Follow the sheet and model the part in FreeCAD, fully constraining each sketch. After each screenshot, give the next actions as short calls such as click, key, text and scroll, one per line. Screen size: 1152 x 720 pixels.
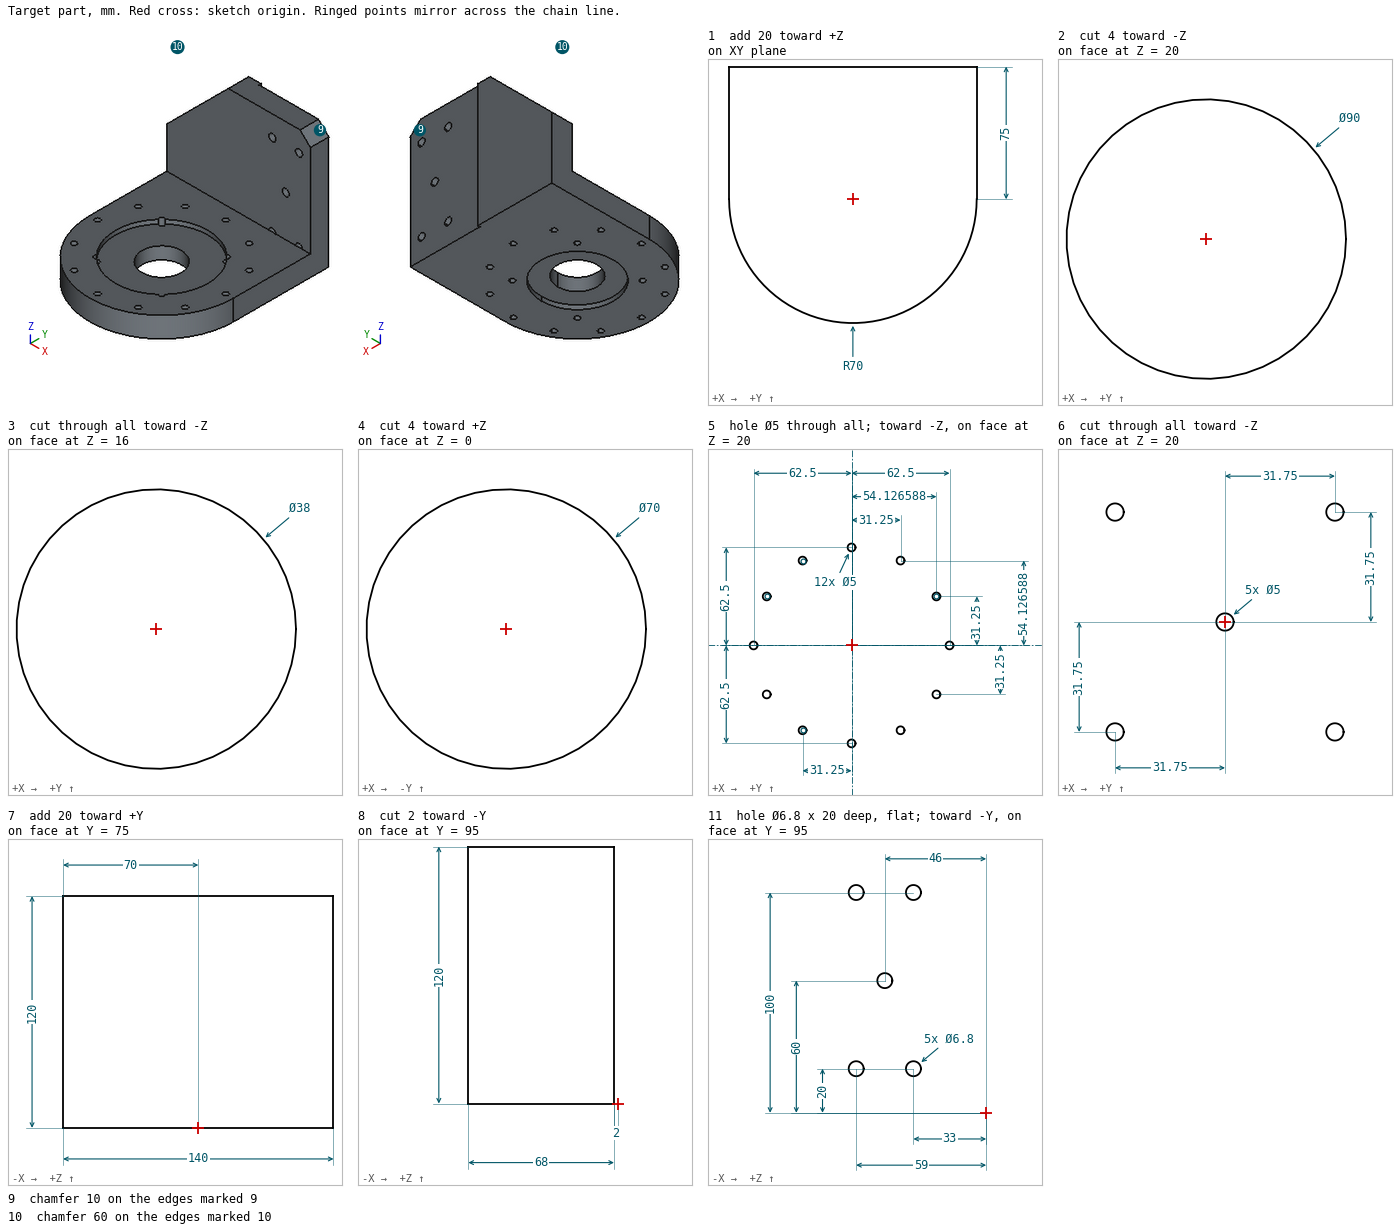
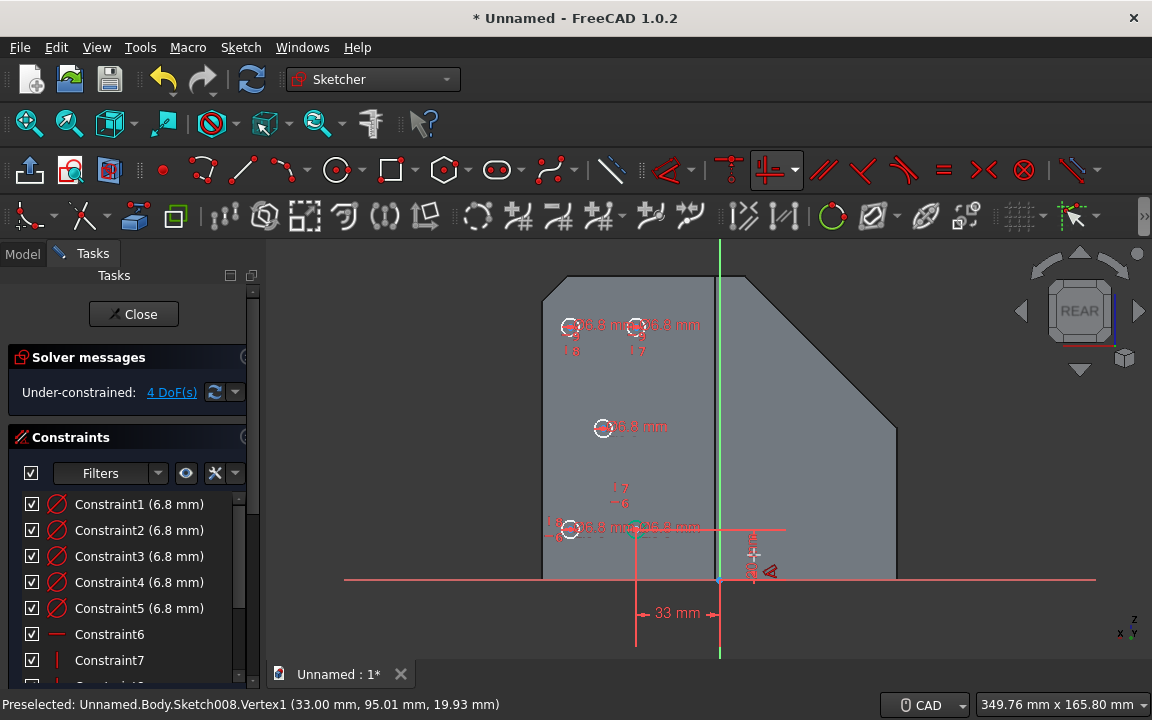
click(570, 530)
click(593, 614)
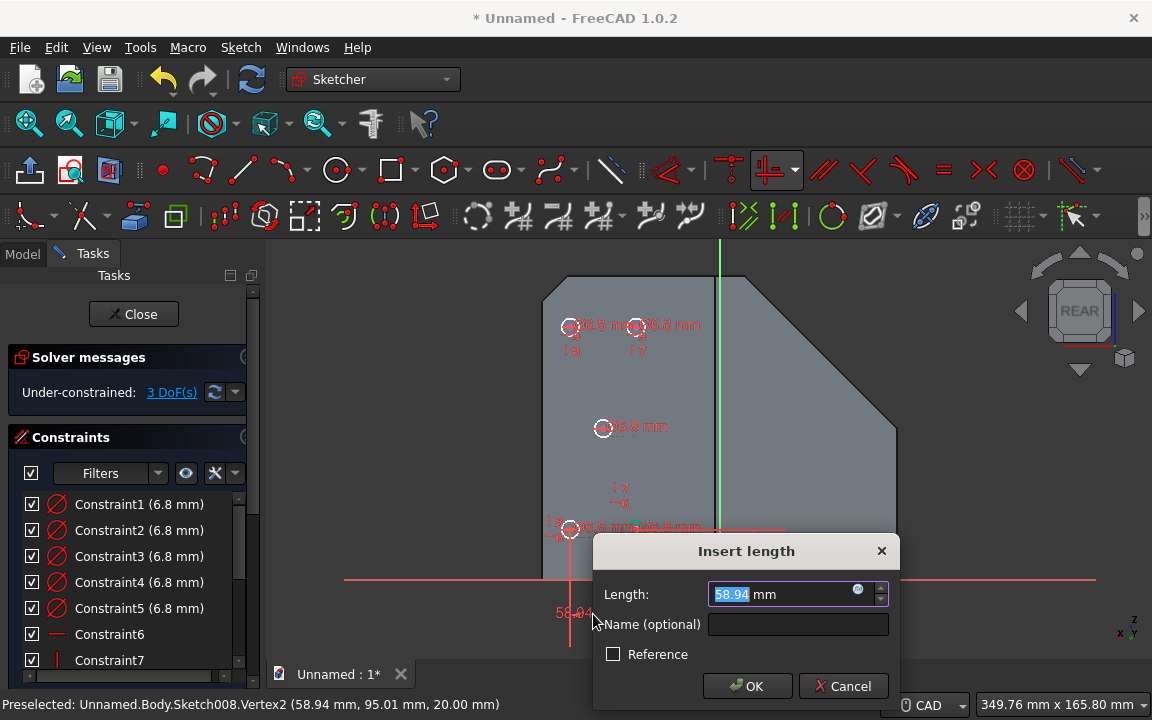
text(59)
key(Return)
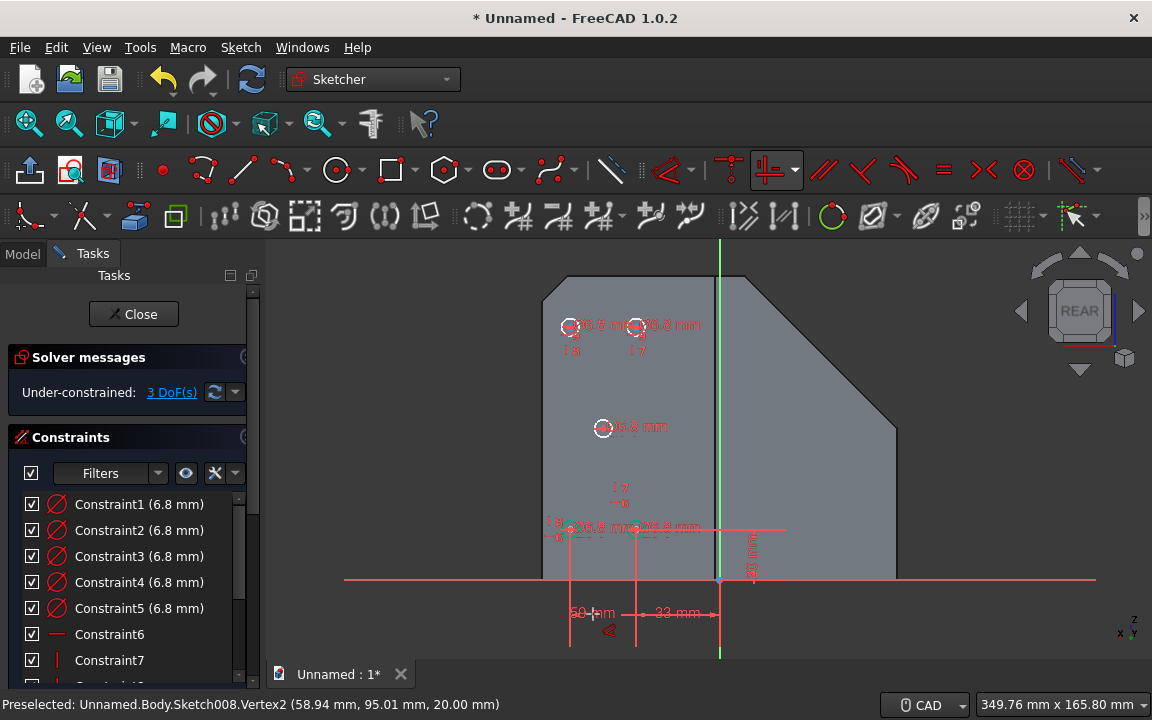
click(603, 429)
click(661, 395)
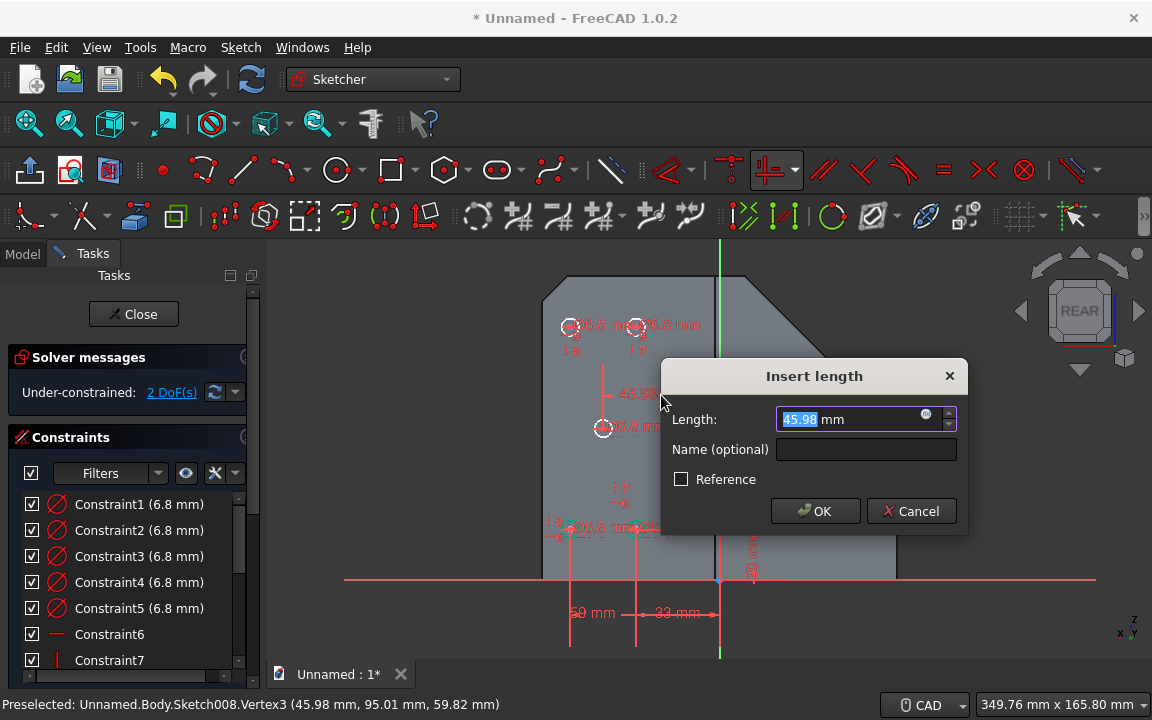
text(46)
key(Return)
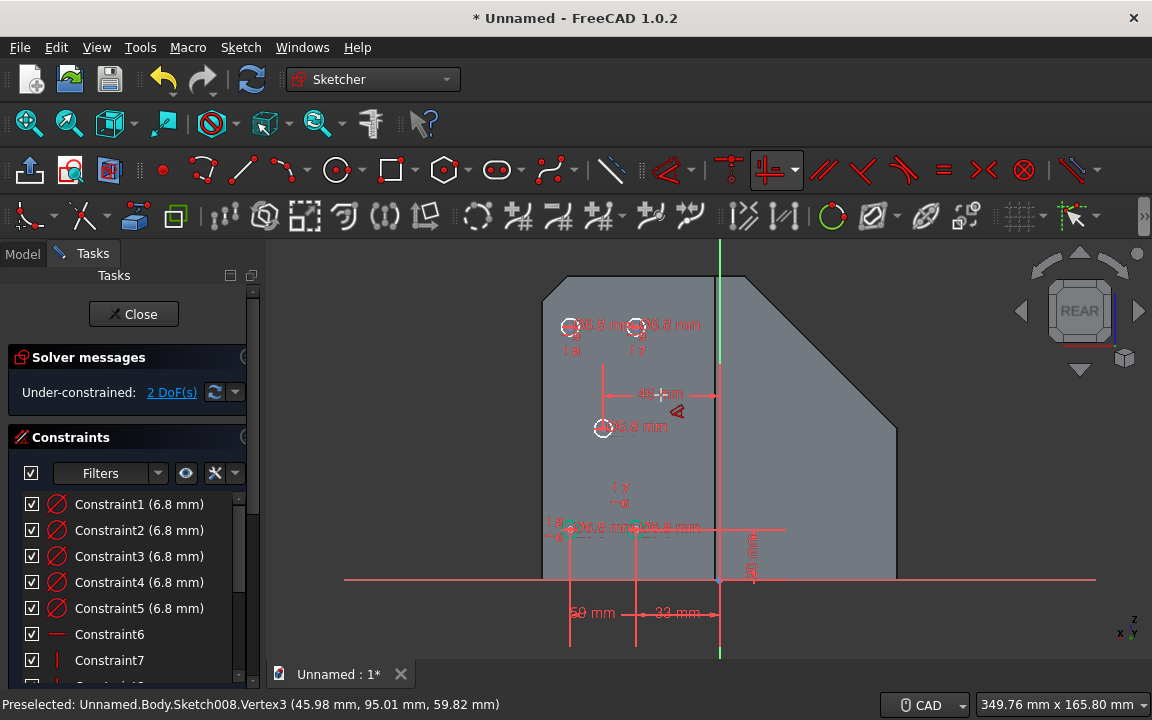
click(603, 429)
click(754, 504)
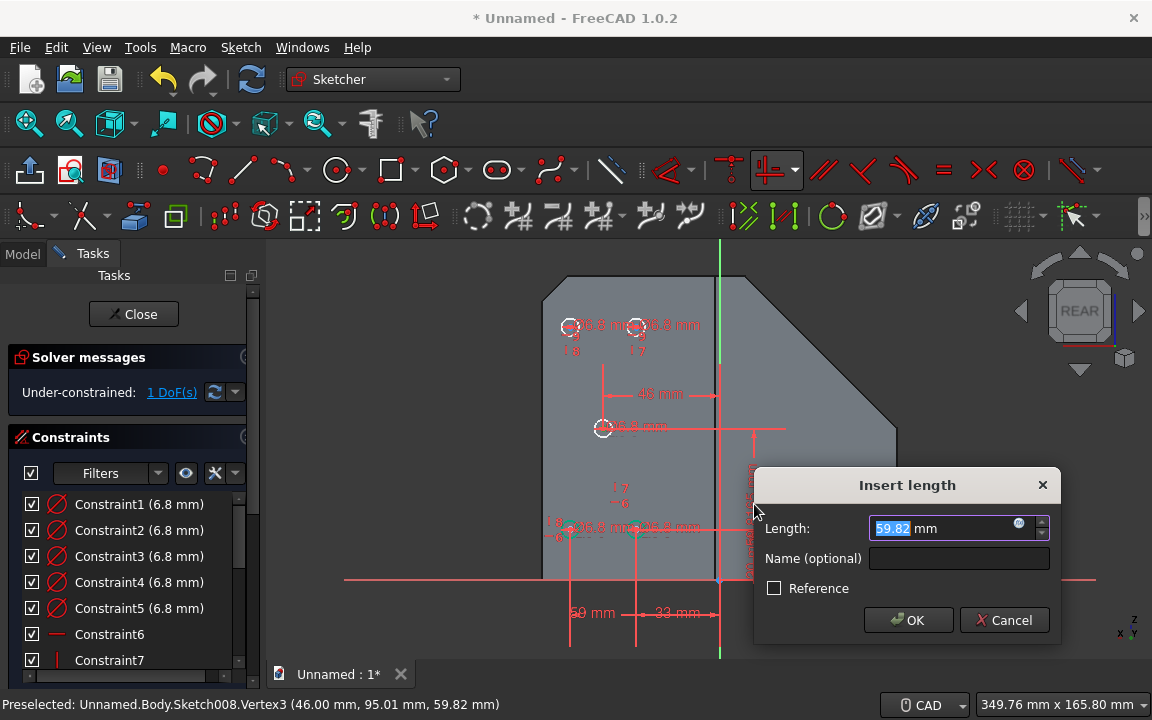
text(60)
key(Return)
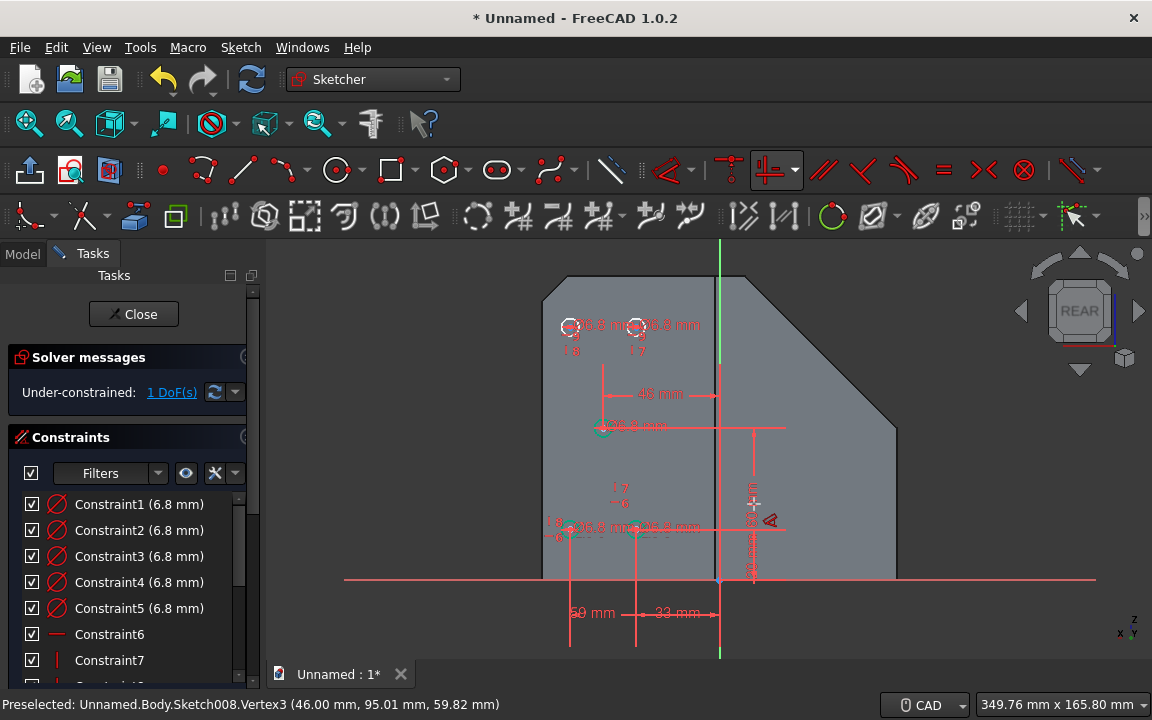
click(636, 327)
click(754, 454)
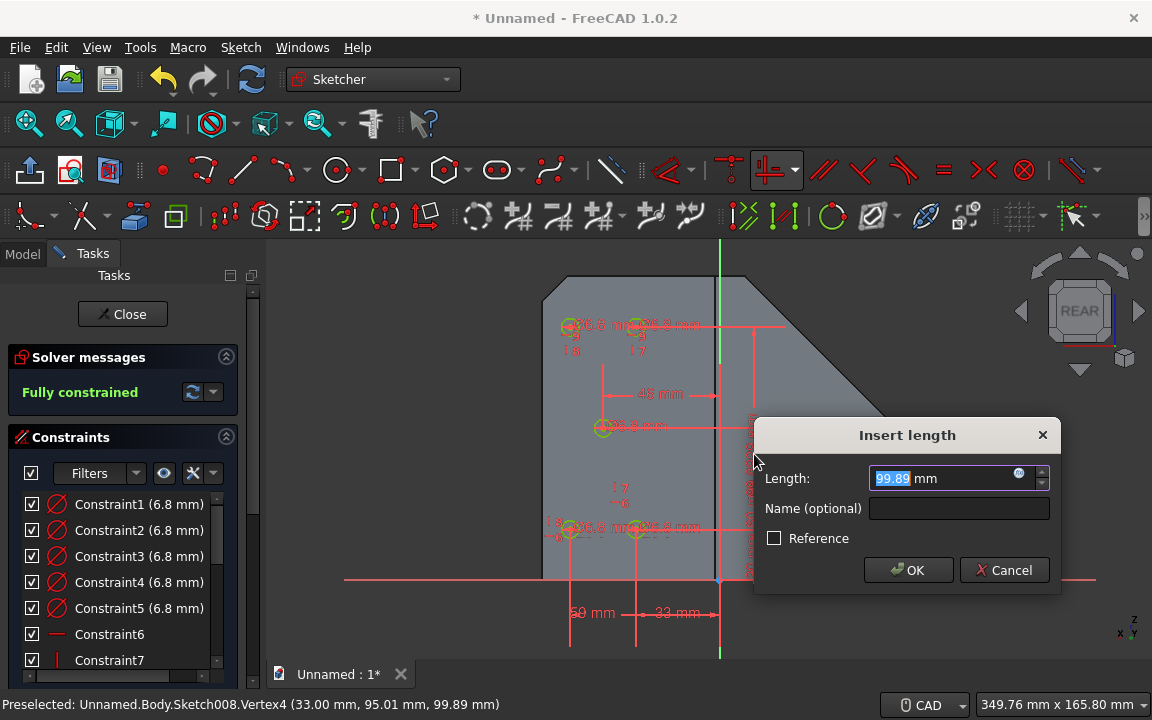
text(100)
key(Return)
key(Escape)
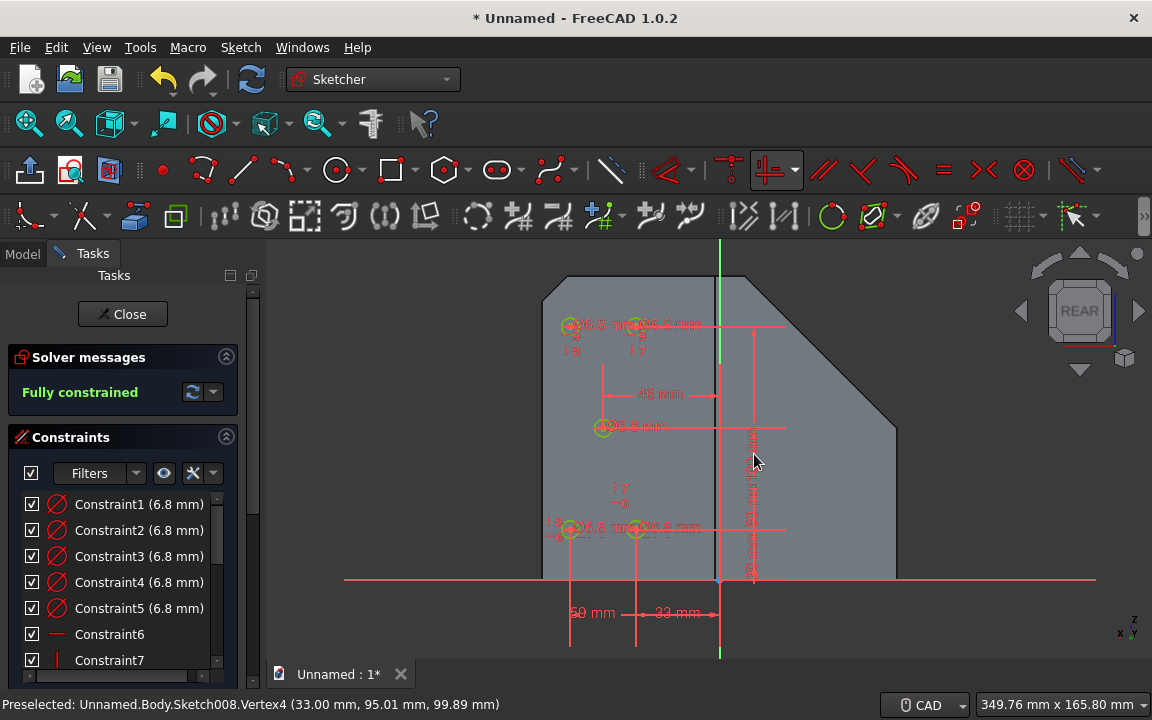
click(123, 314)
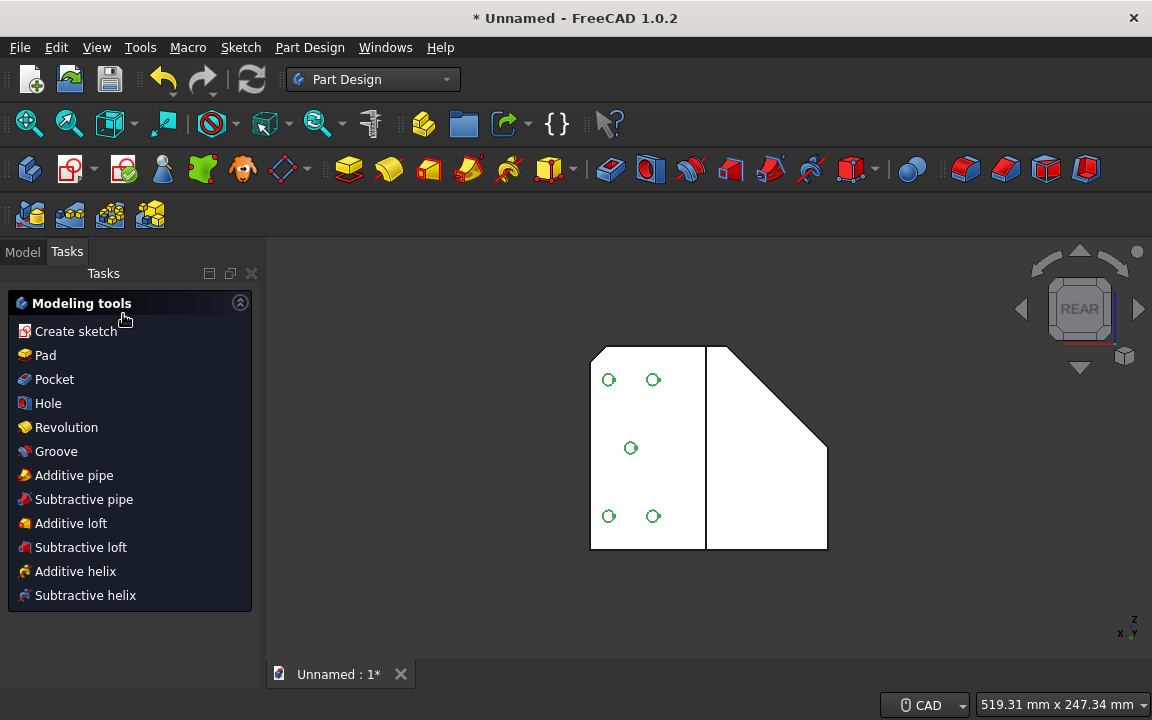
click(652, 170)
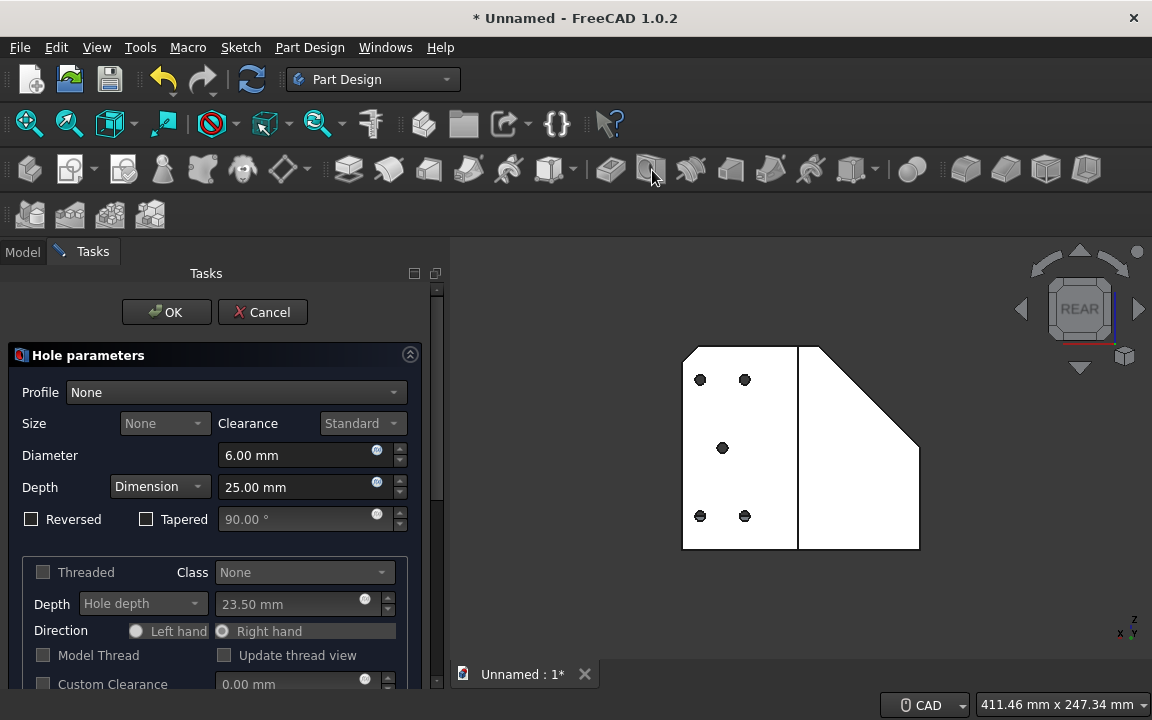
triple_click(305, 455)